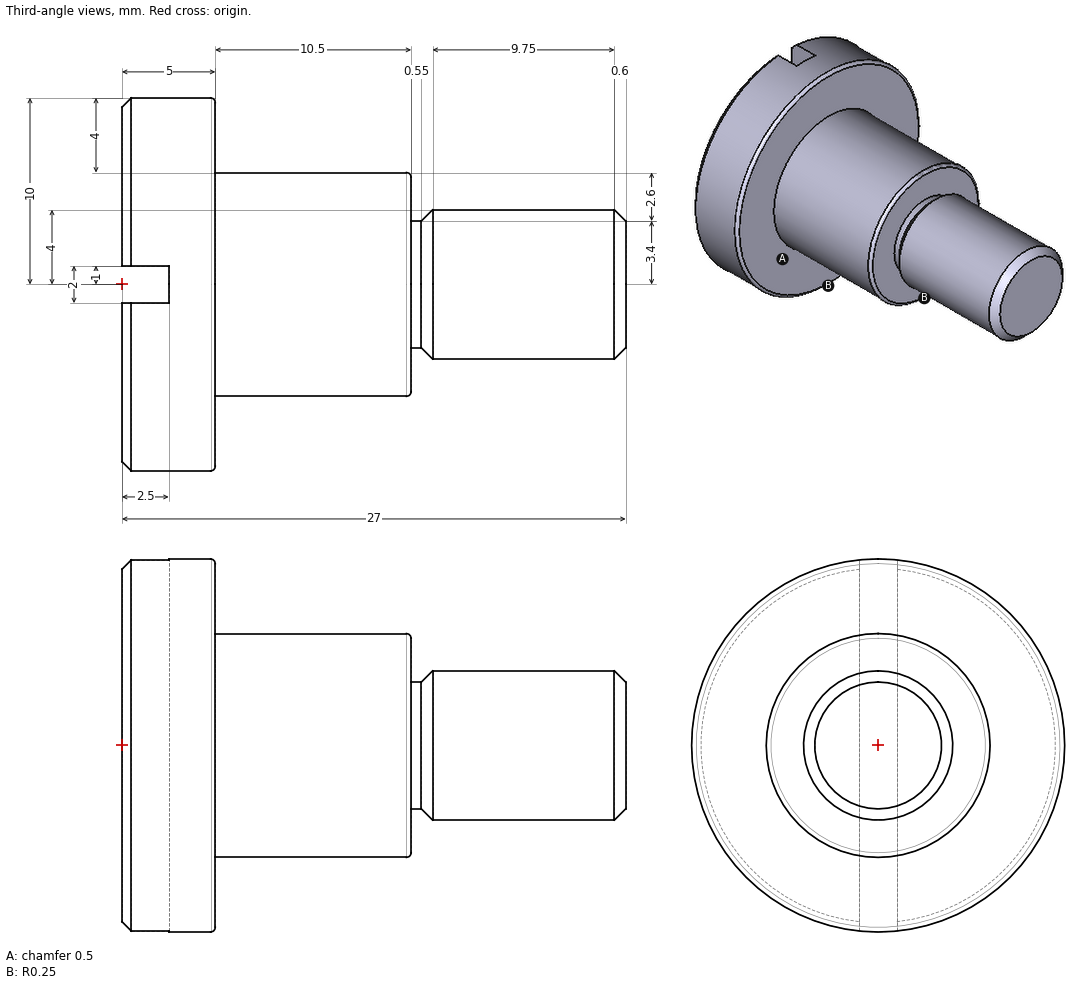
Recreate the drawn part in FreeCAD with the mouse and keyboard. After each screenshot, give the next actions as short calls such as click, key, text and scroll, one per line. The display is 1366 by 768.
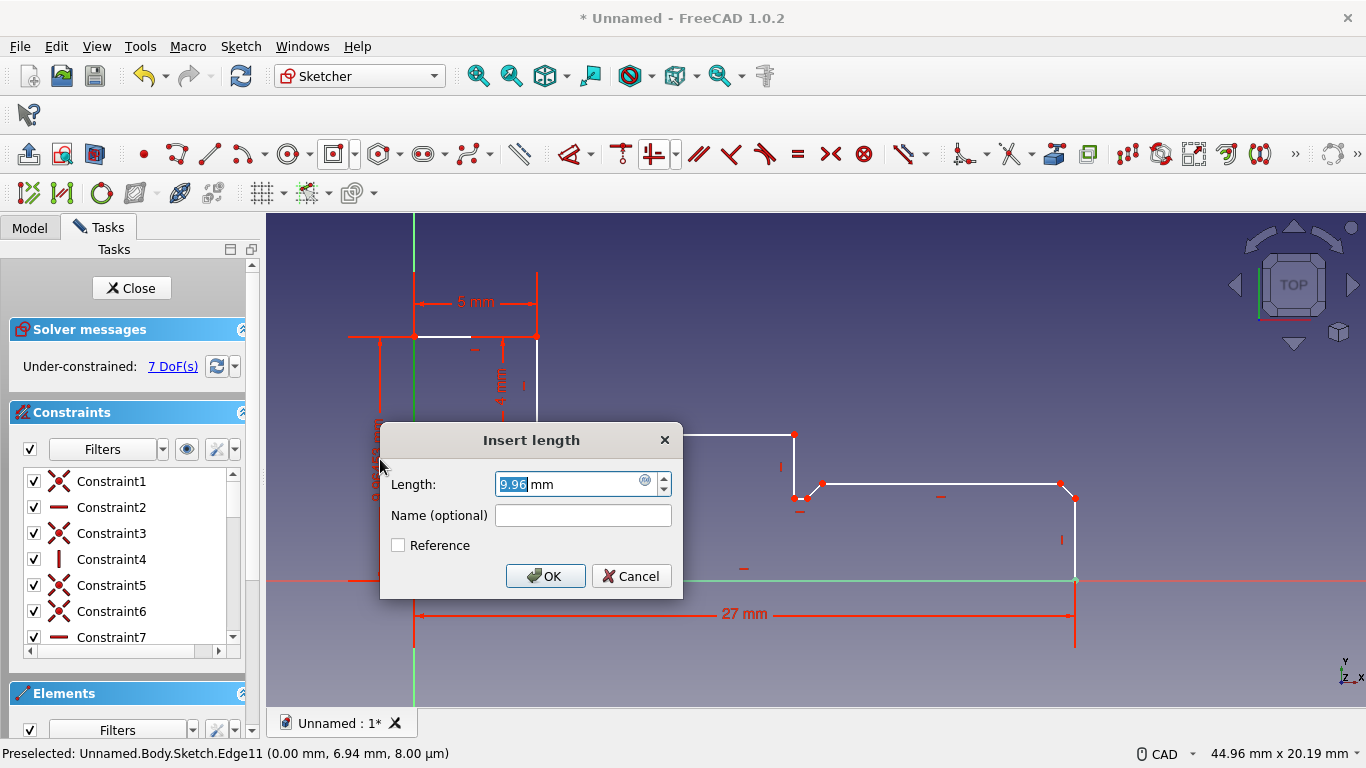
text(10)
key(Return)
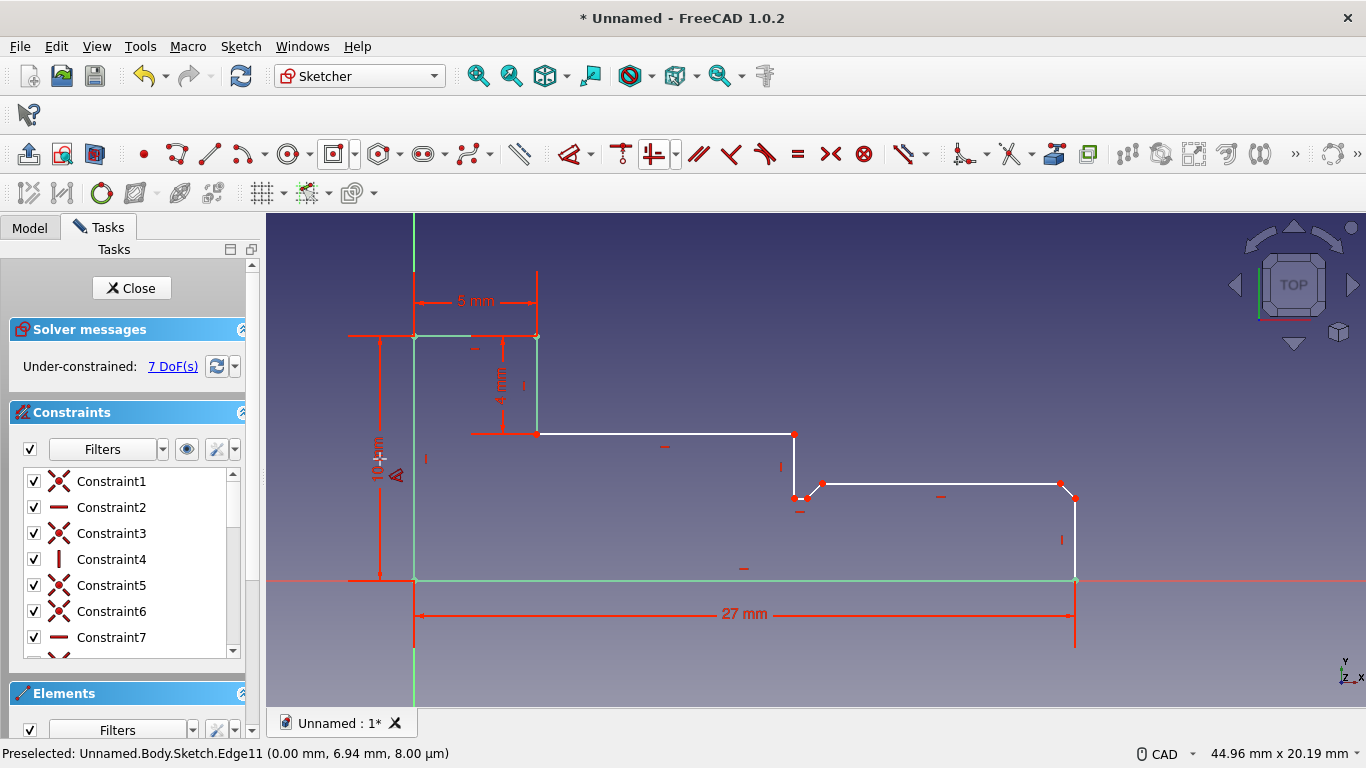
click(1060, 484)
click(380, 532)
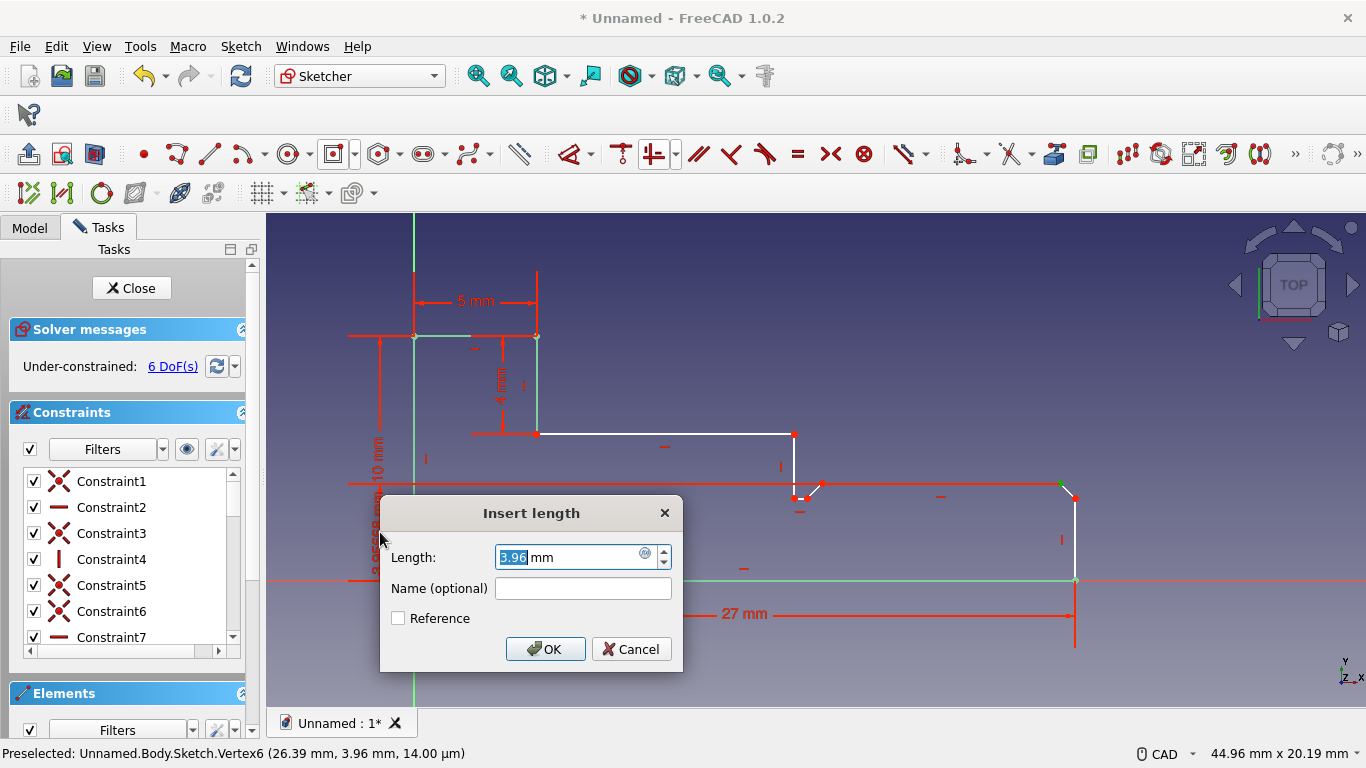
text(4)
key(Return)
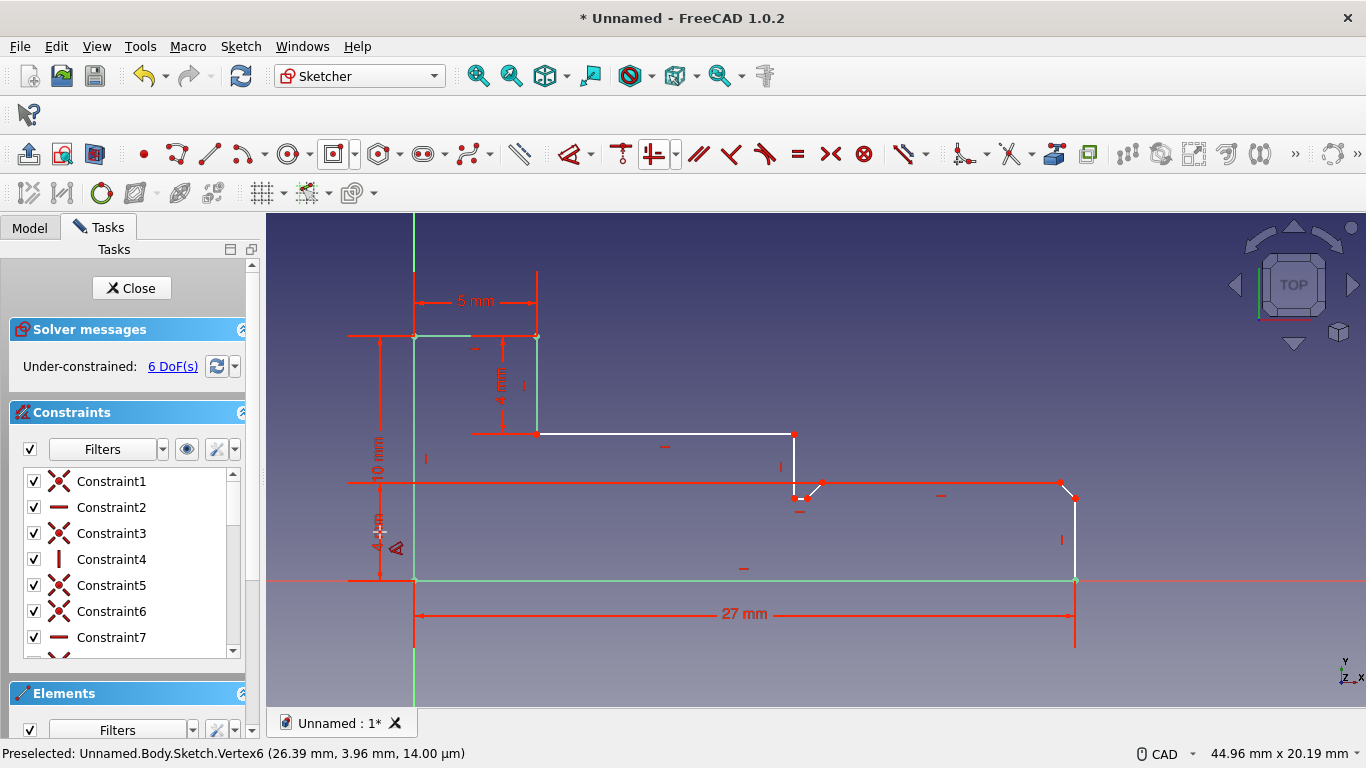
click(1075, 556)
click(1109, 540)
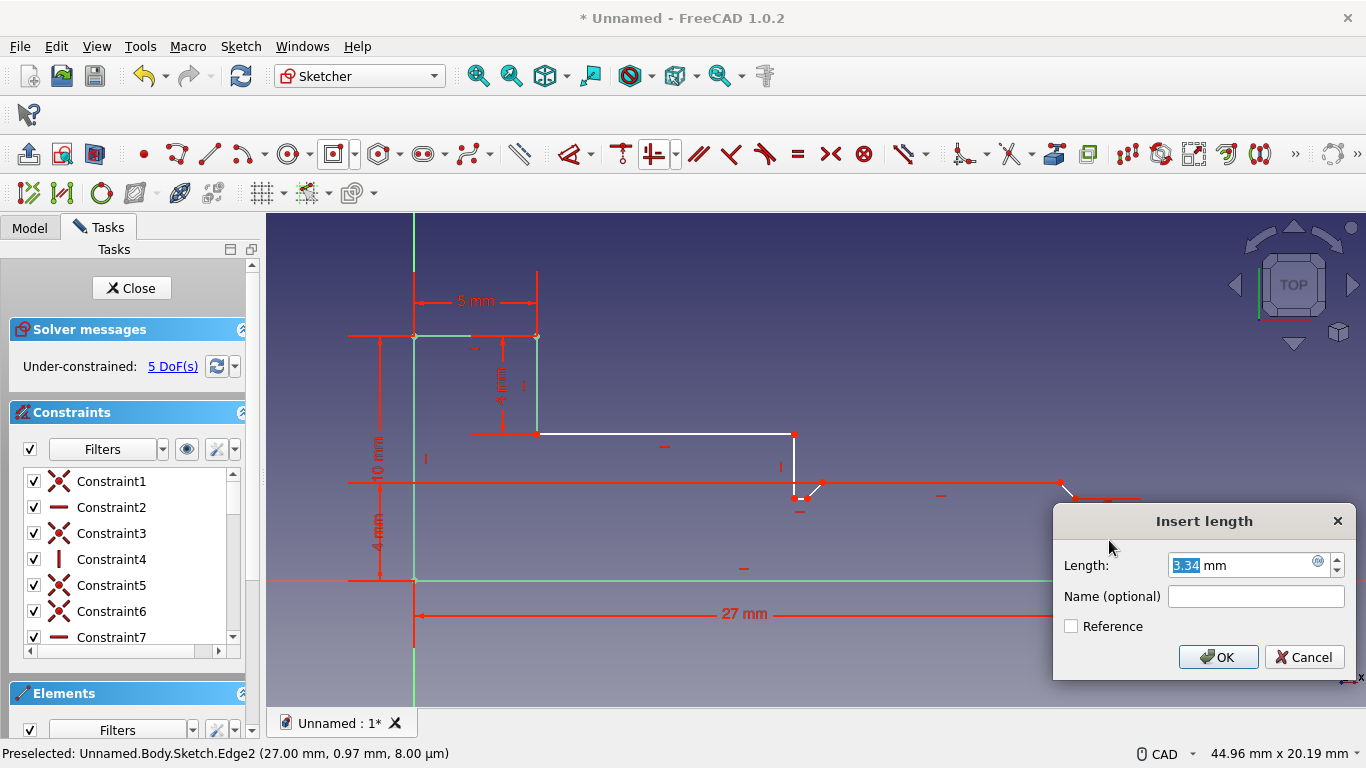
text(3.4)
key(Return)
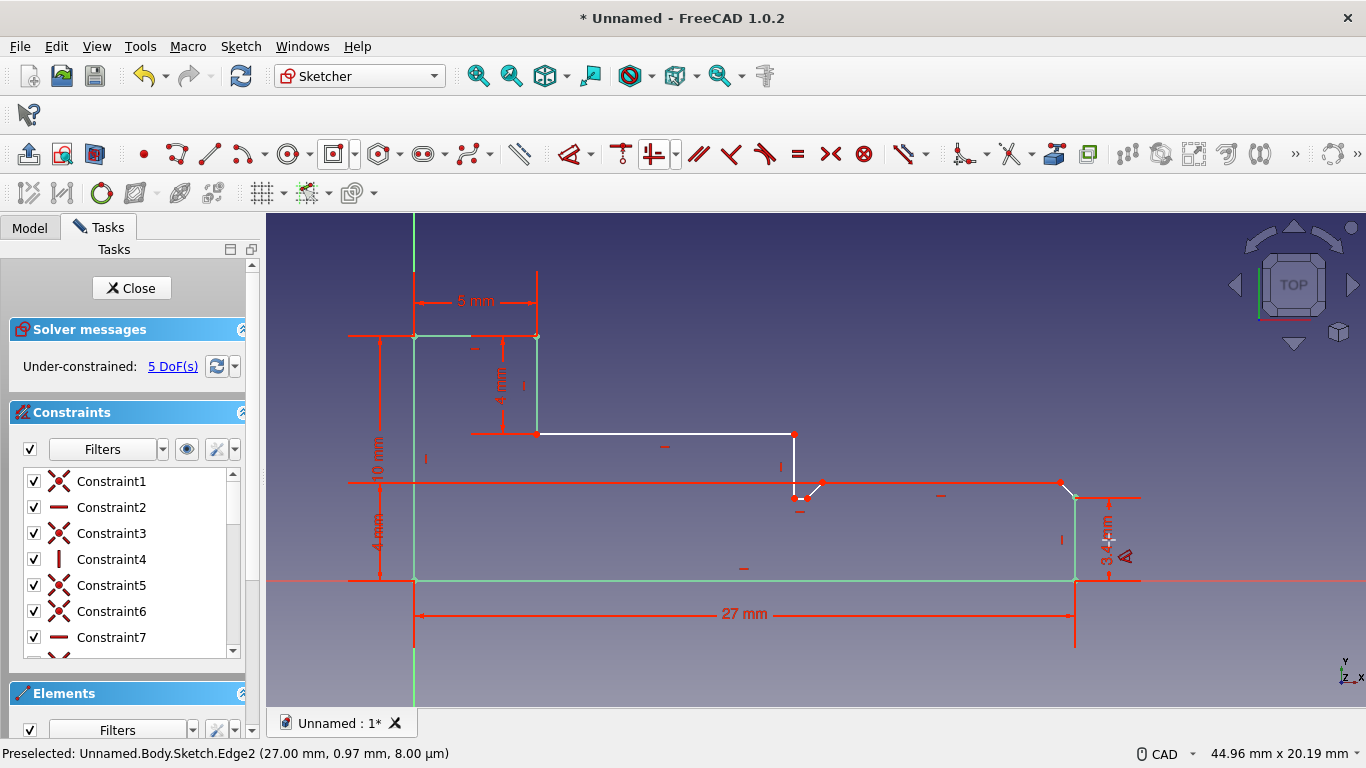
click(794, 480)
click(828, 467)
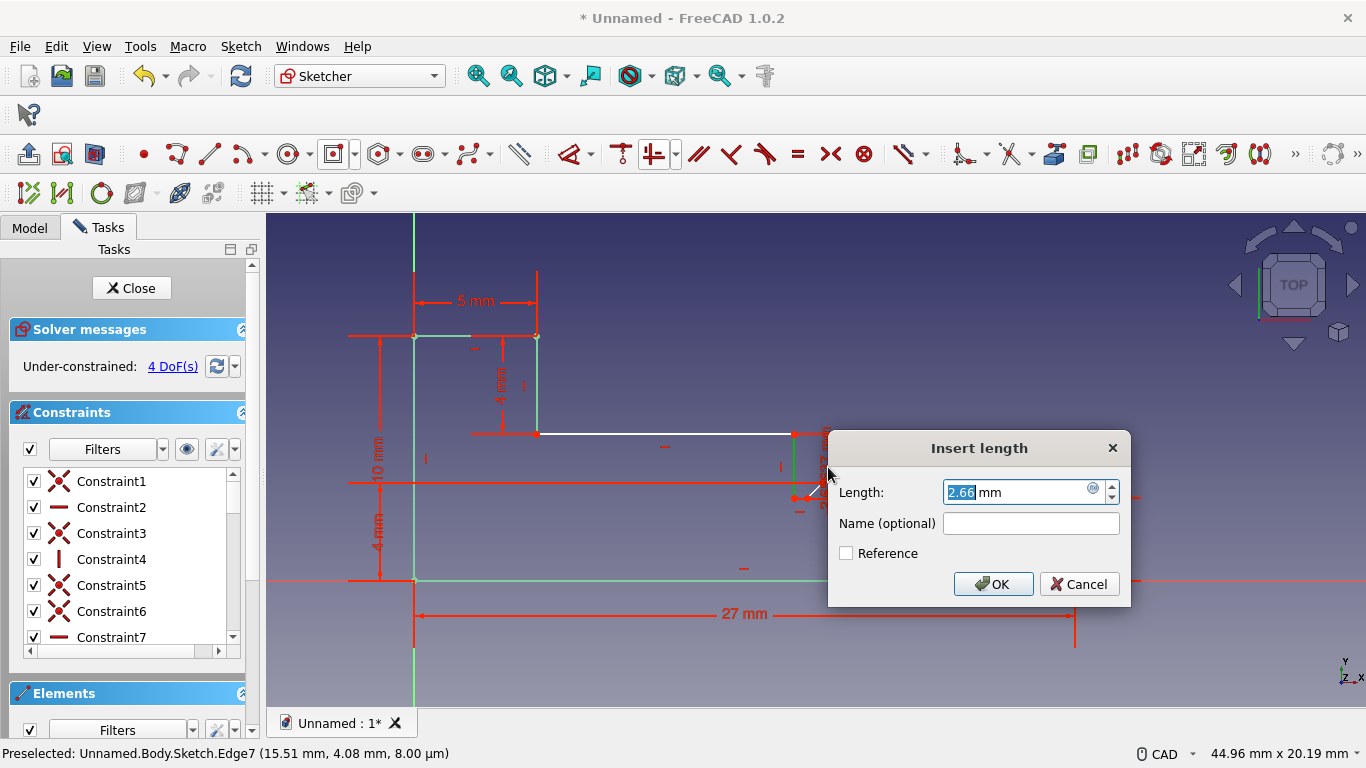
text(2.6)
key(Return)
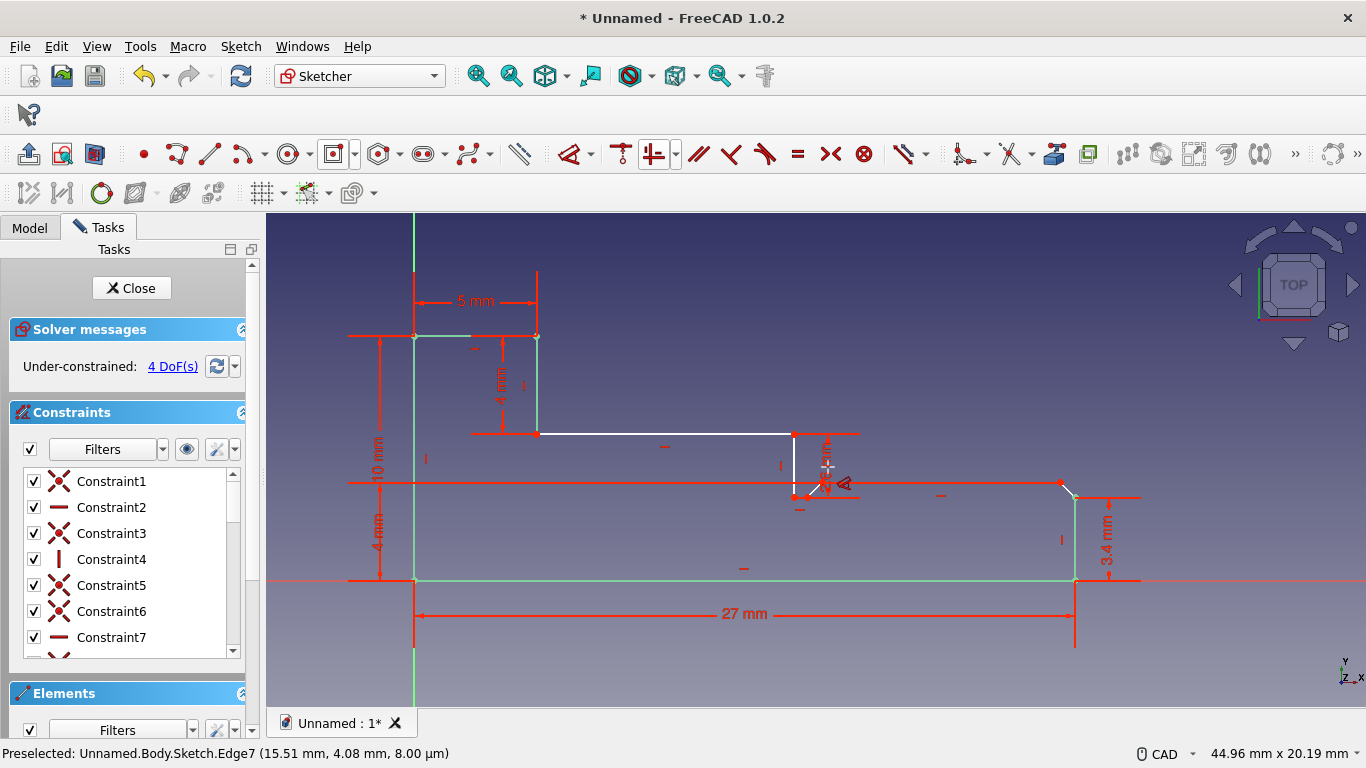
click(989, 483)
click(941, 517)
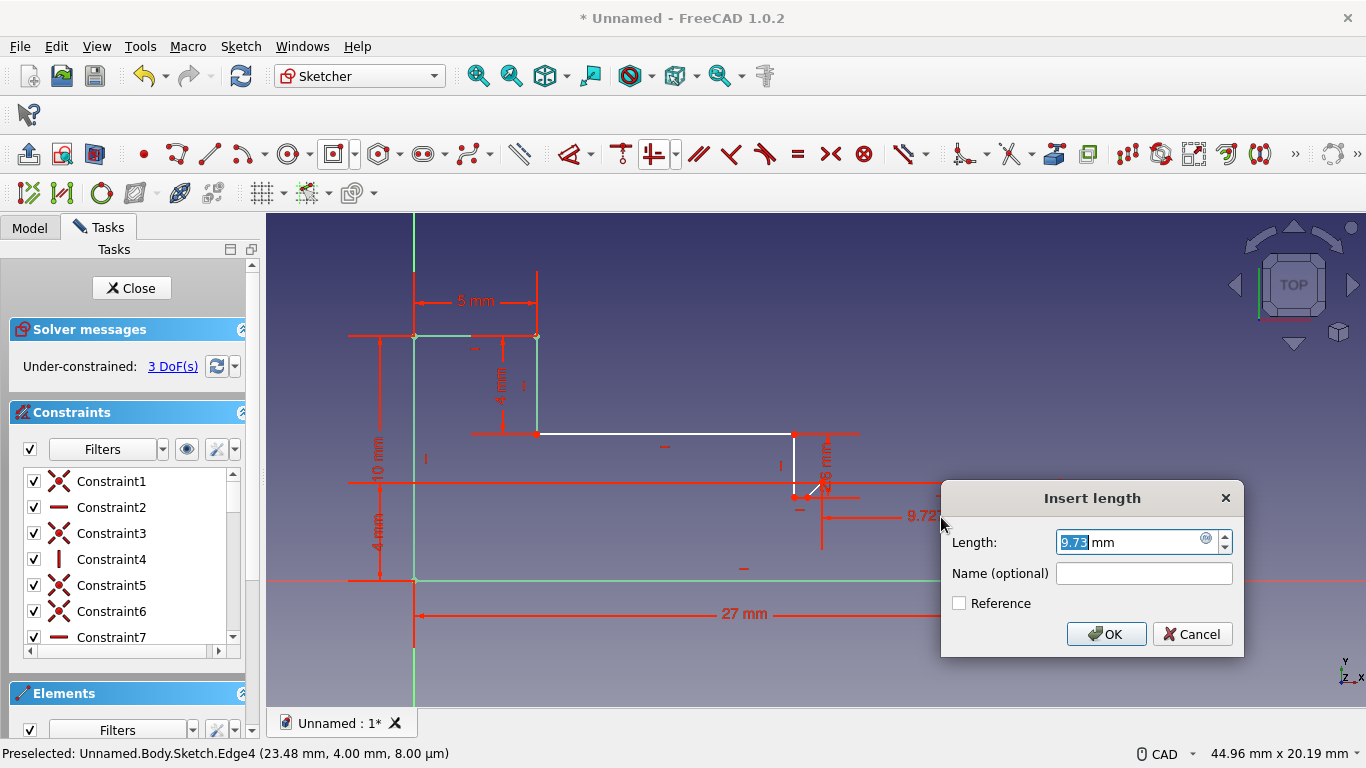
text(9.75)
key(Return)